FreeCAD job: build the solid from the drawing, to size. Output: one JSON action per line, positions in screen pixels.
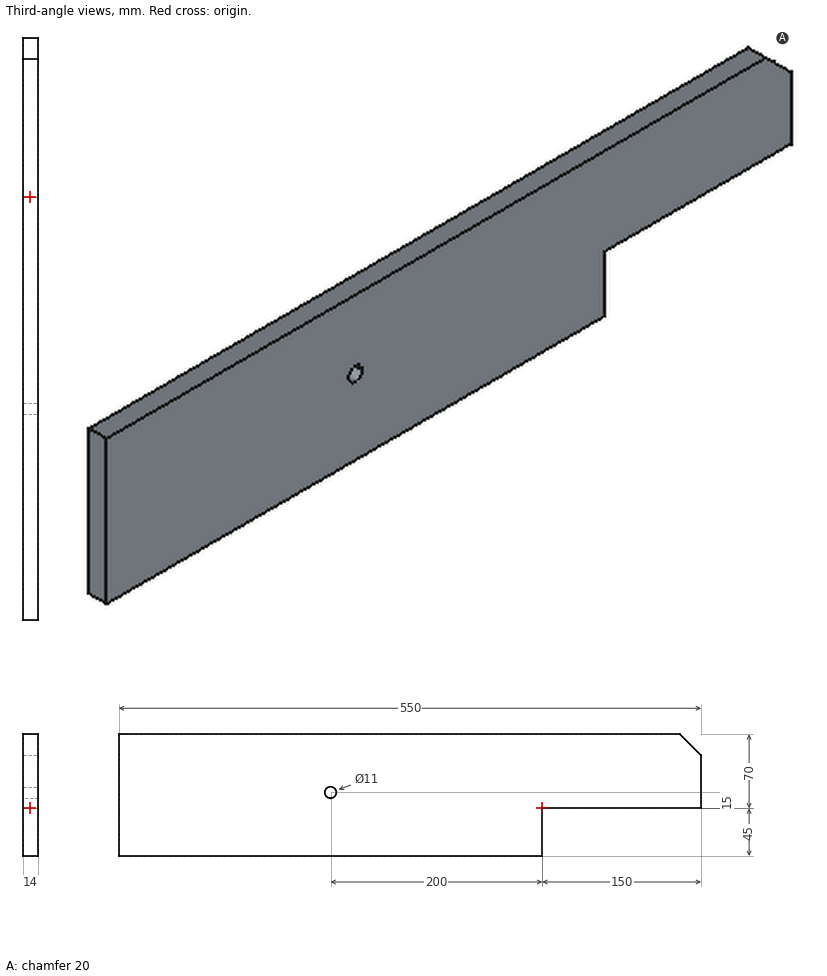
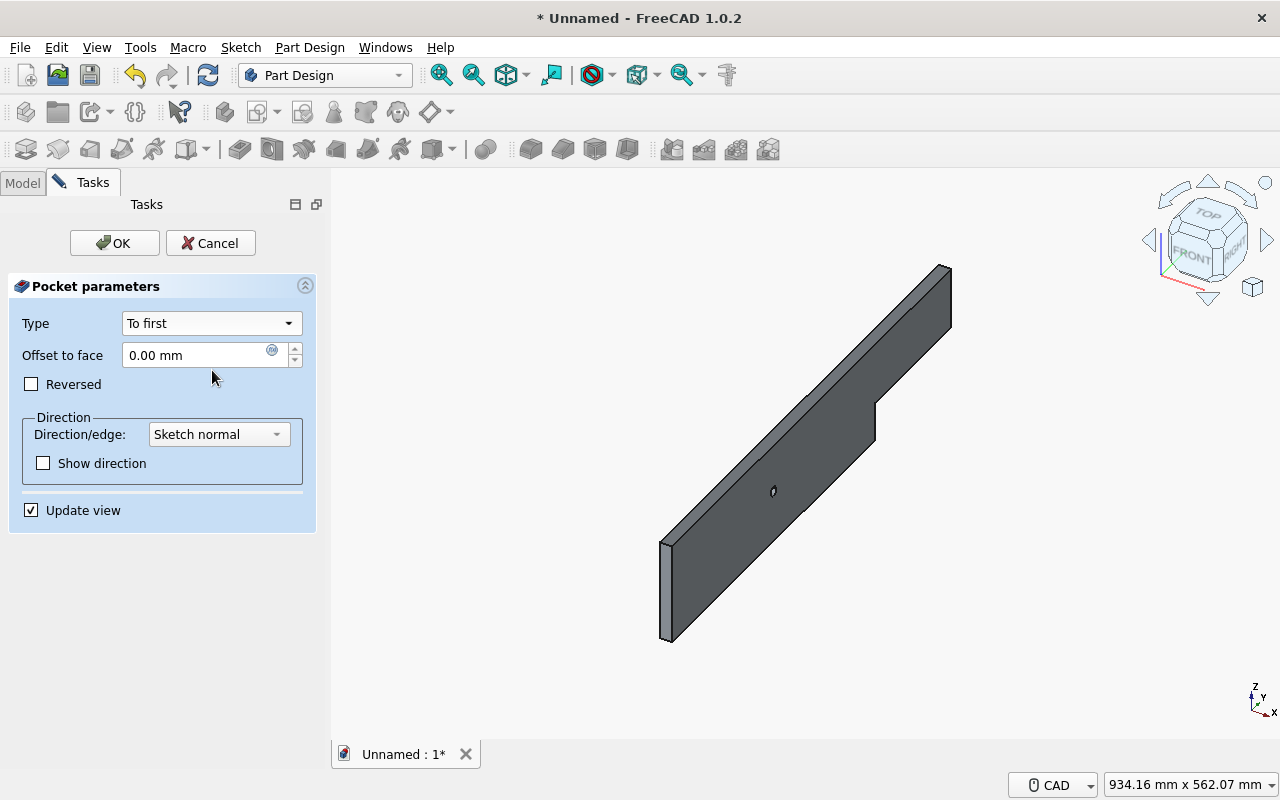
{"action": "left_click", "coordinate": [115, 243]}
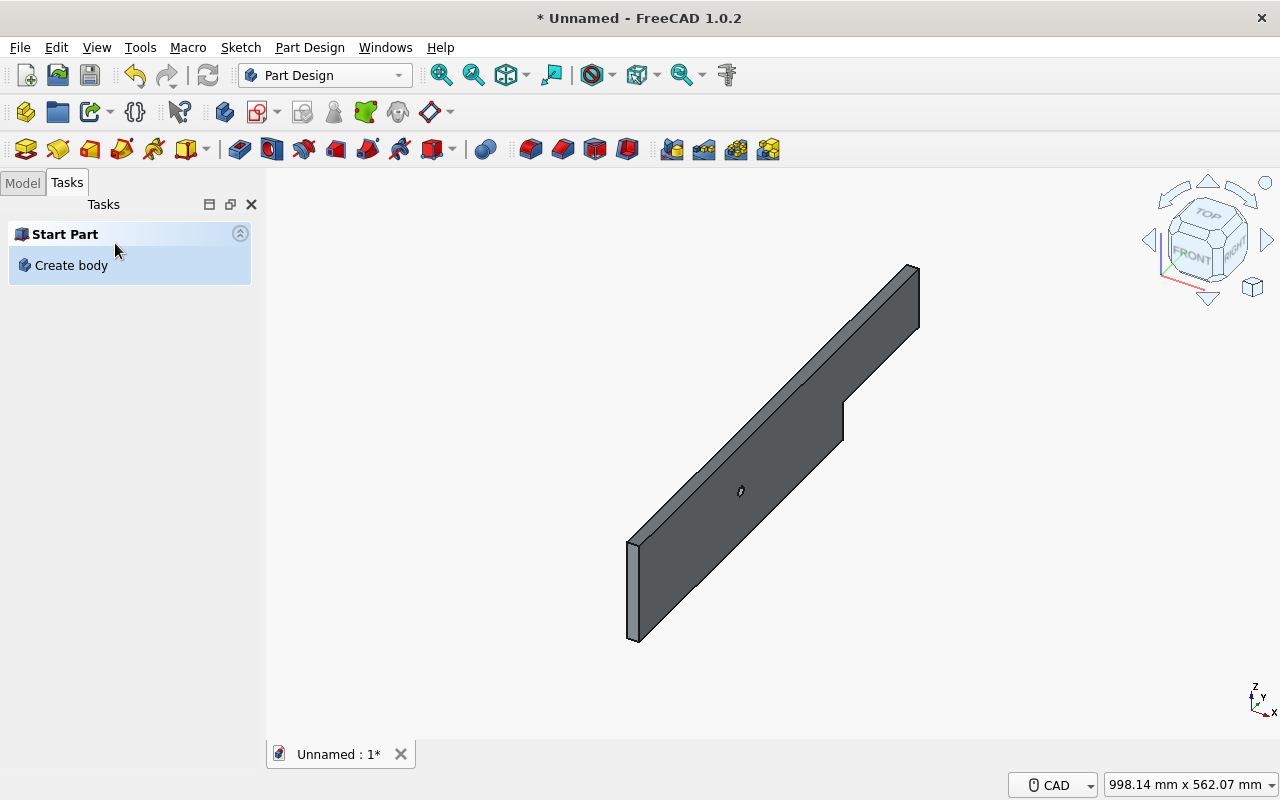
{"action": "scroll", "coordinate": [913, 266], "scroll_direction": "up", "scroll_amount": 6}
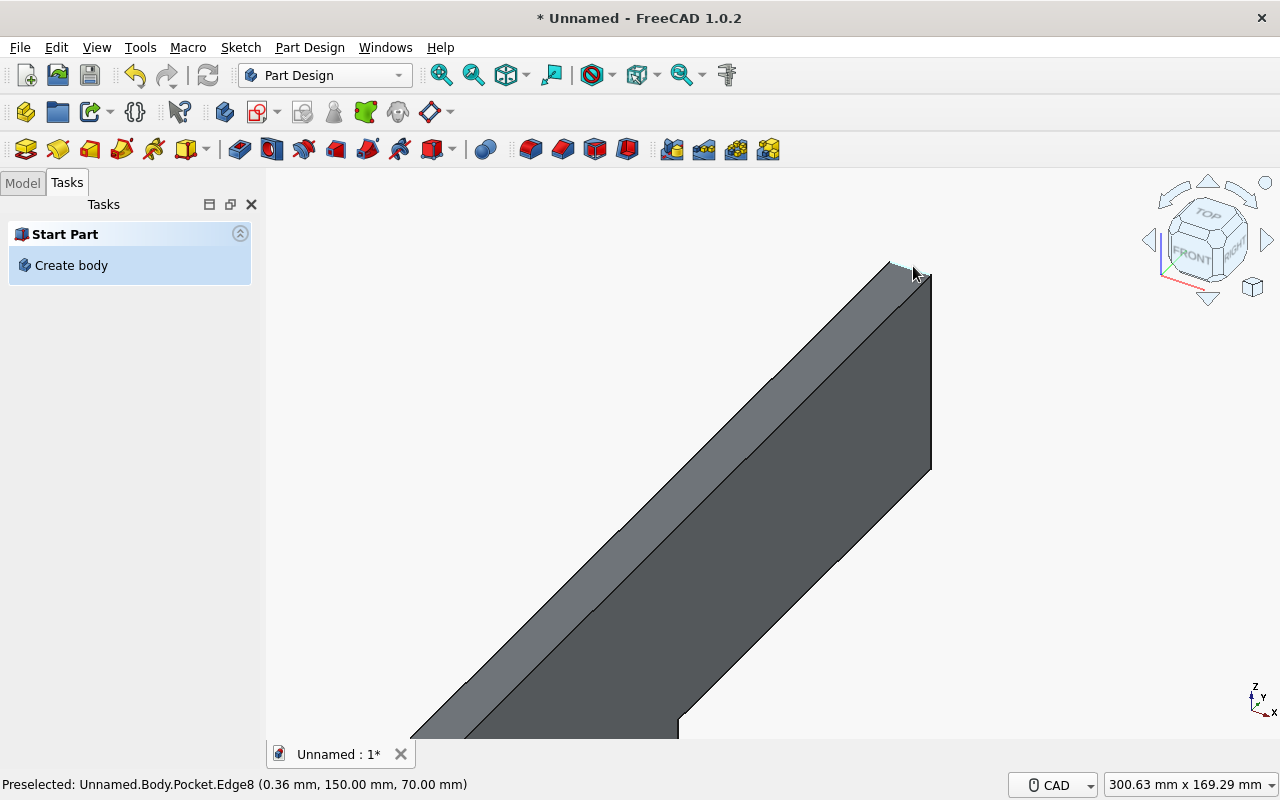
{"action": "left_click", "coordinate": [442, 76]}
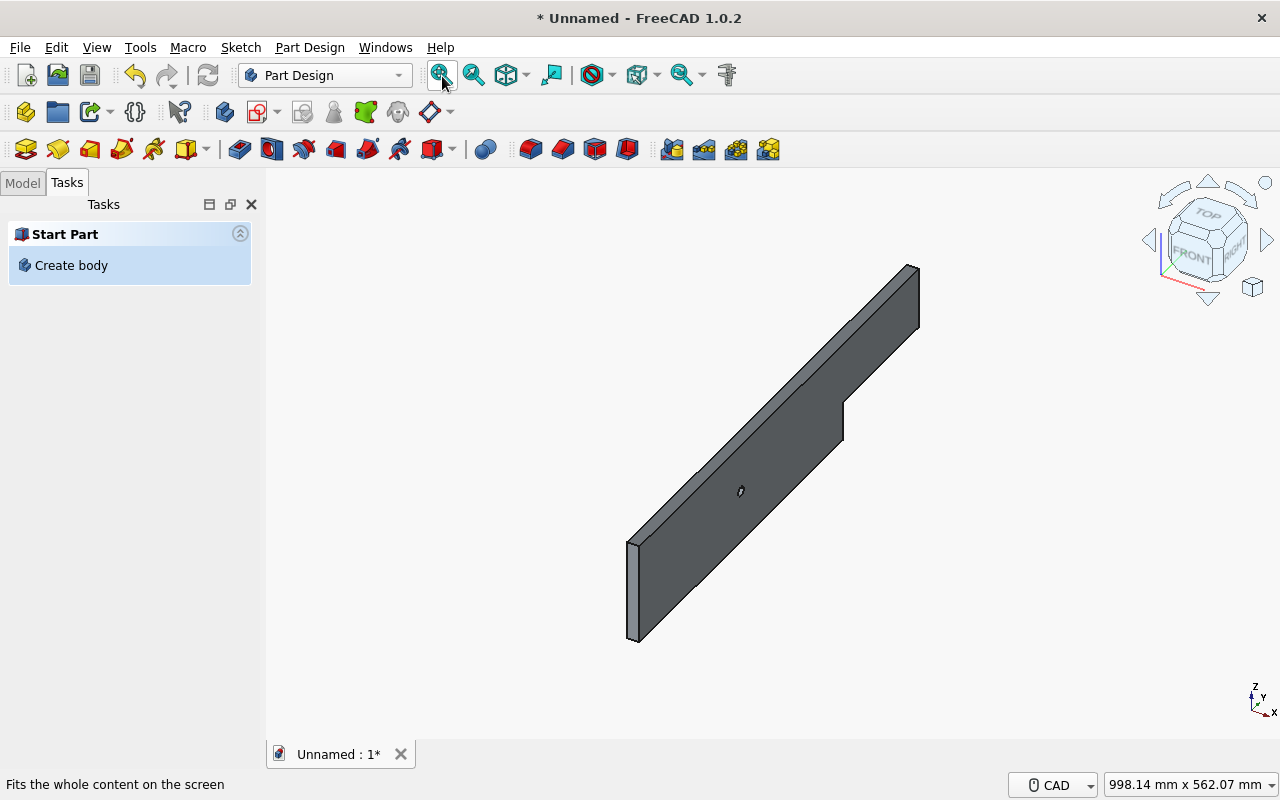
{"action": "key", "text": "0"}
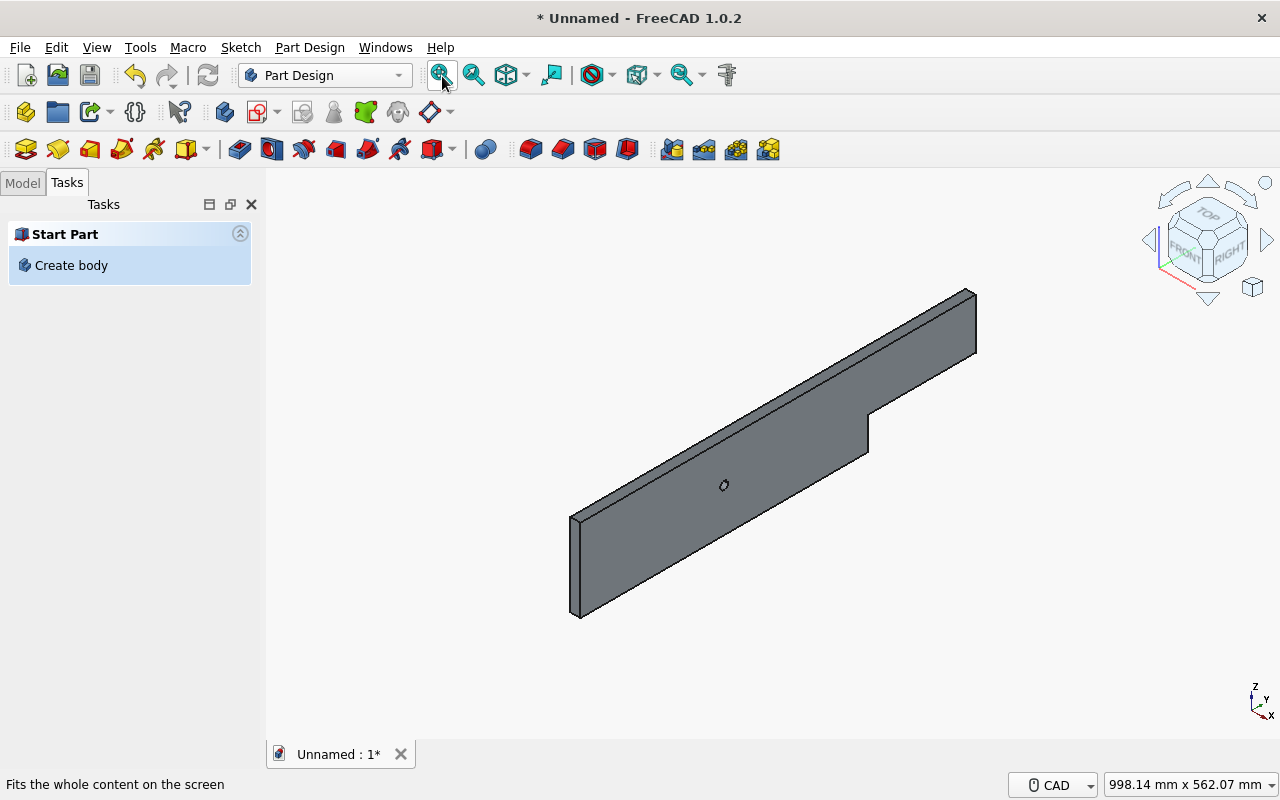
{"action": "scroll", "coordinate": [971, 291], "scroll_direction": "up", "scroll_amount": 6}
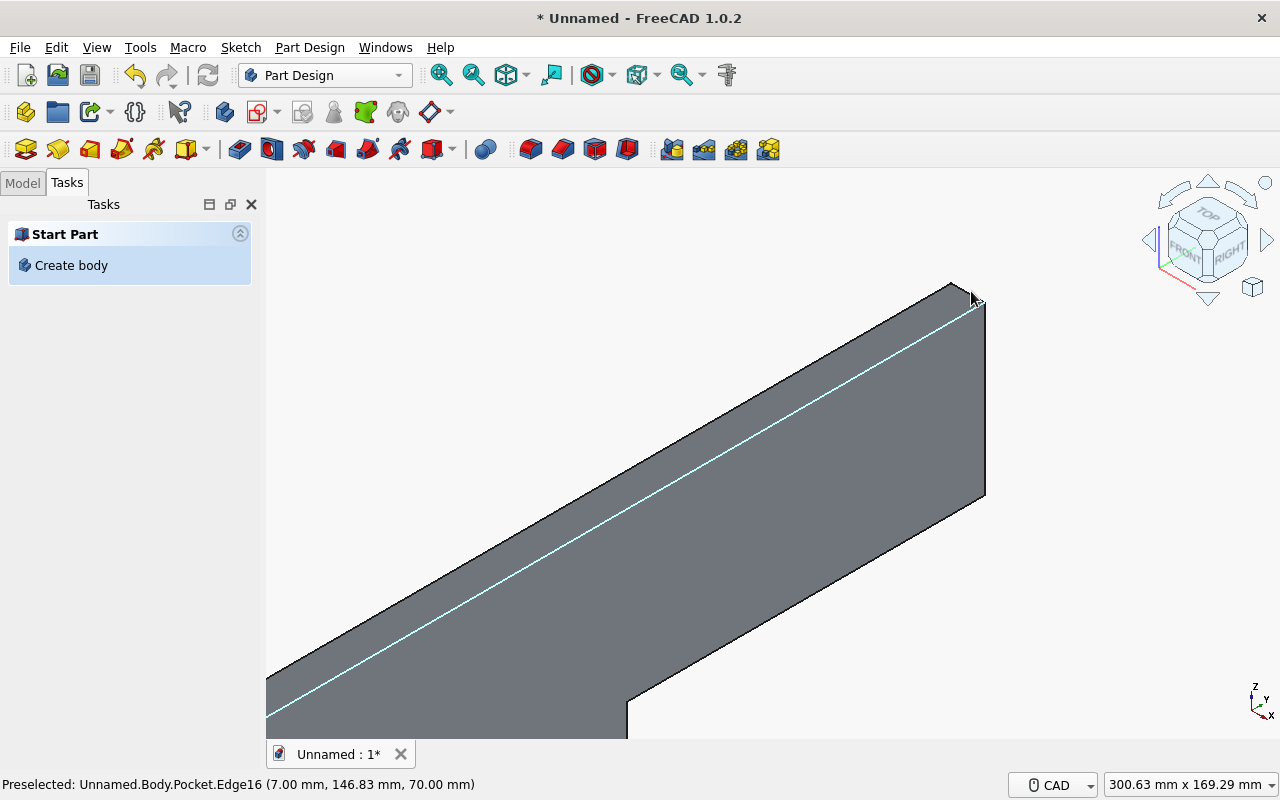
{"action": "left_click", "coordinate": [442, 76]}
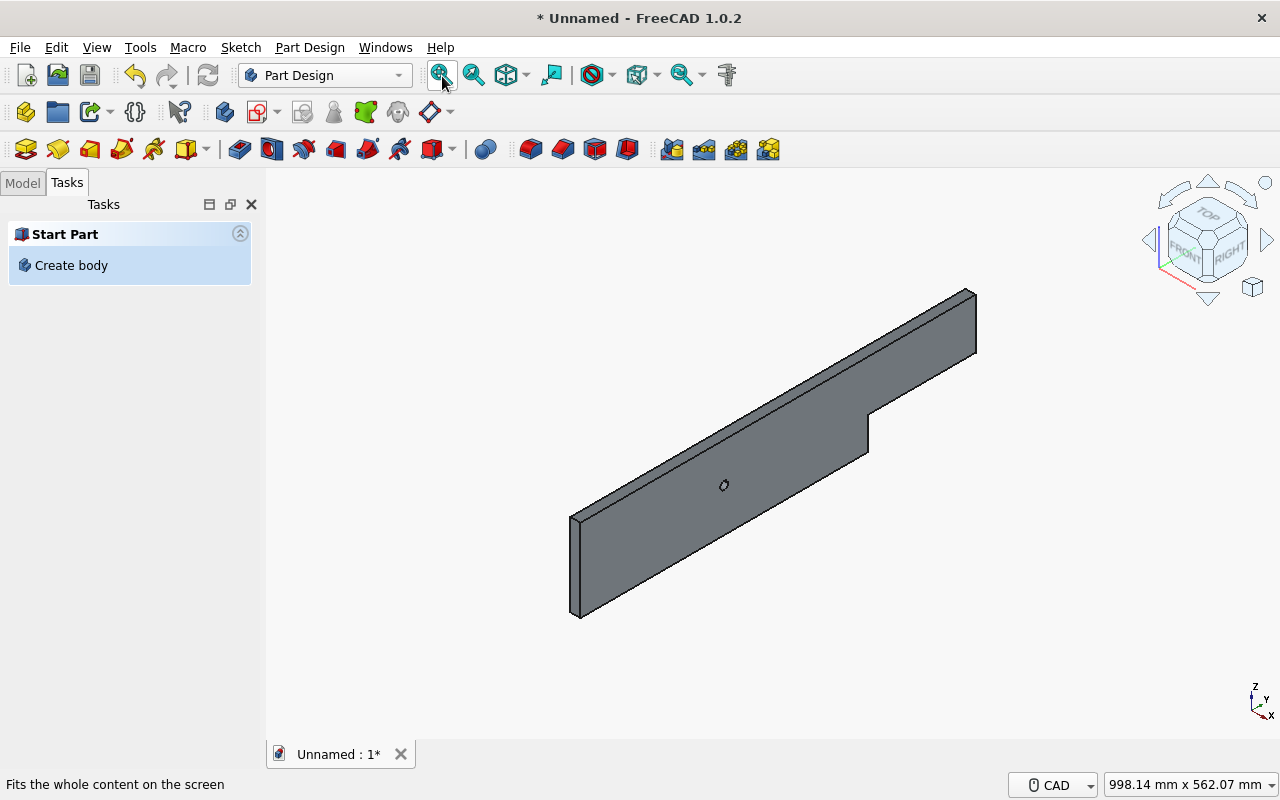
{"action": "key", "text": "2"}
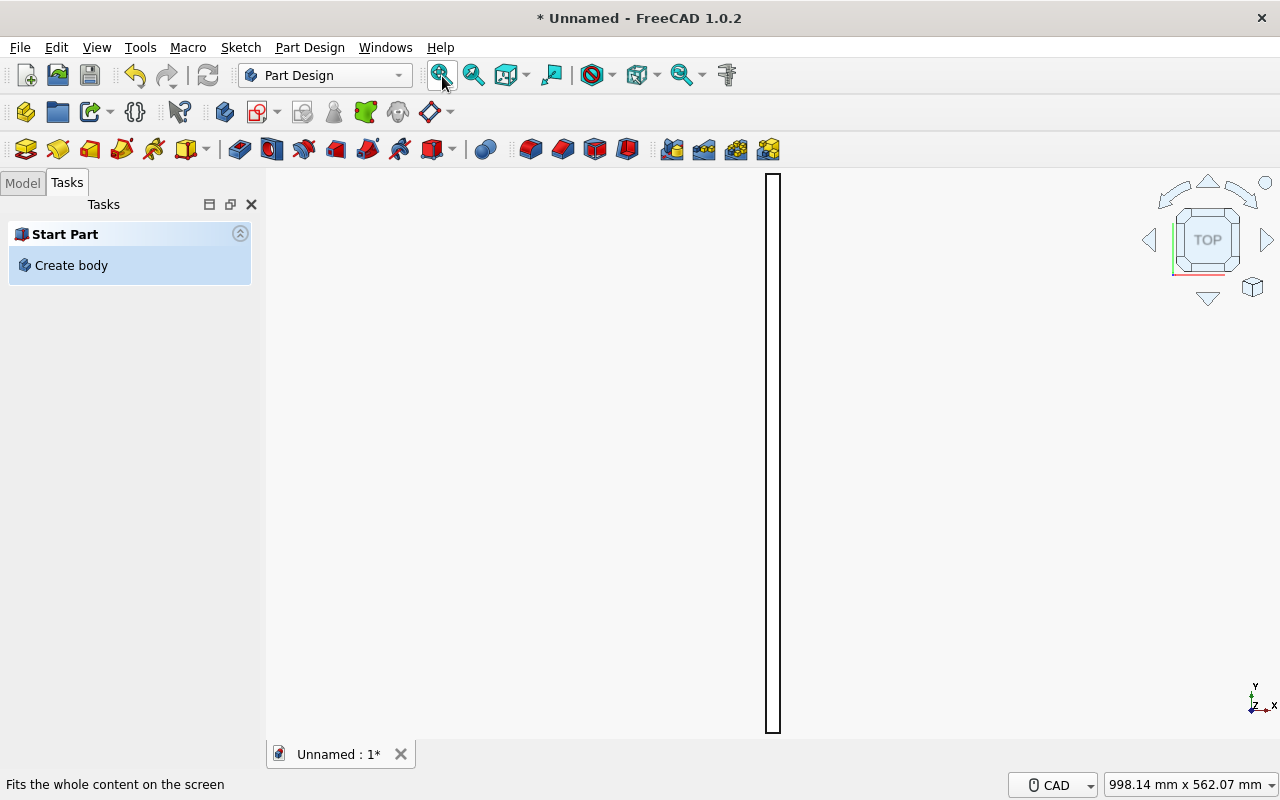
{"action": "key", "text": "1"}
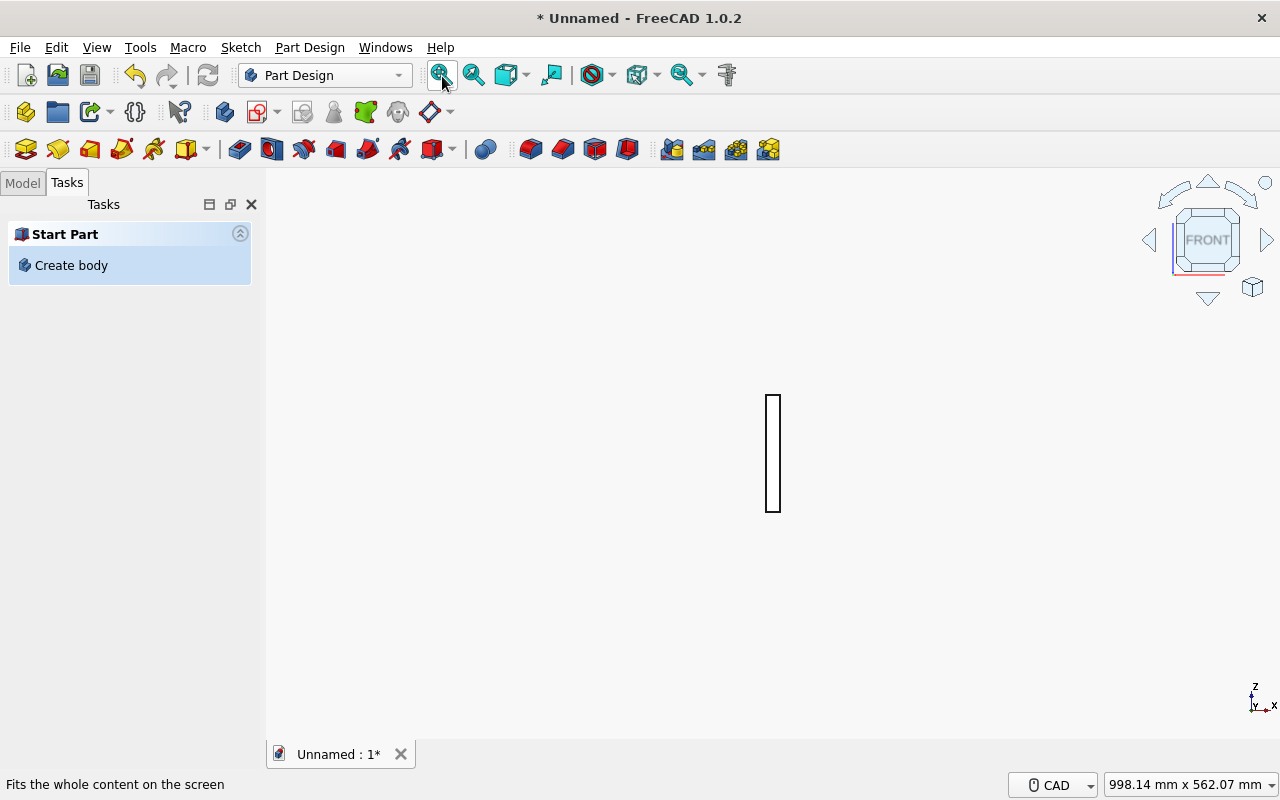
{"action": "left_click", "coordinate": [442, 76]}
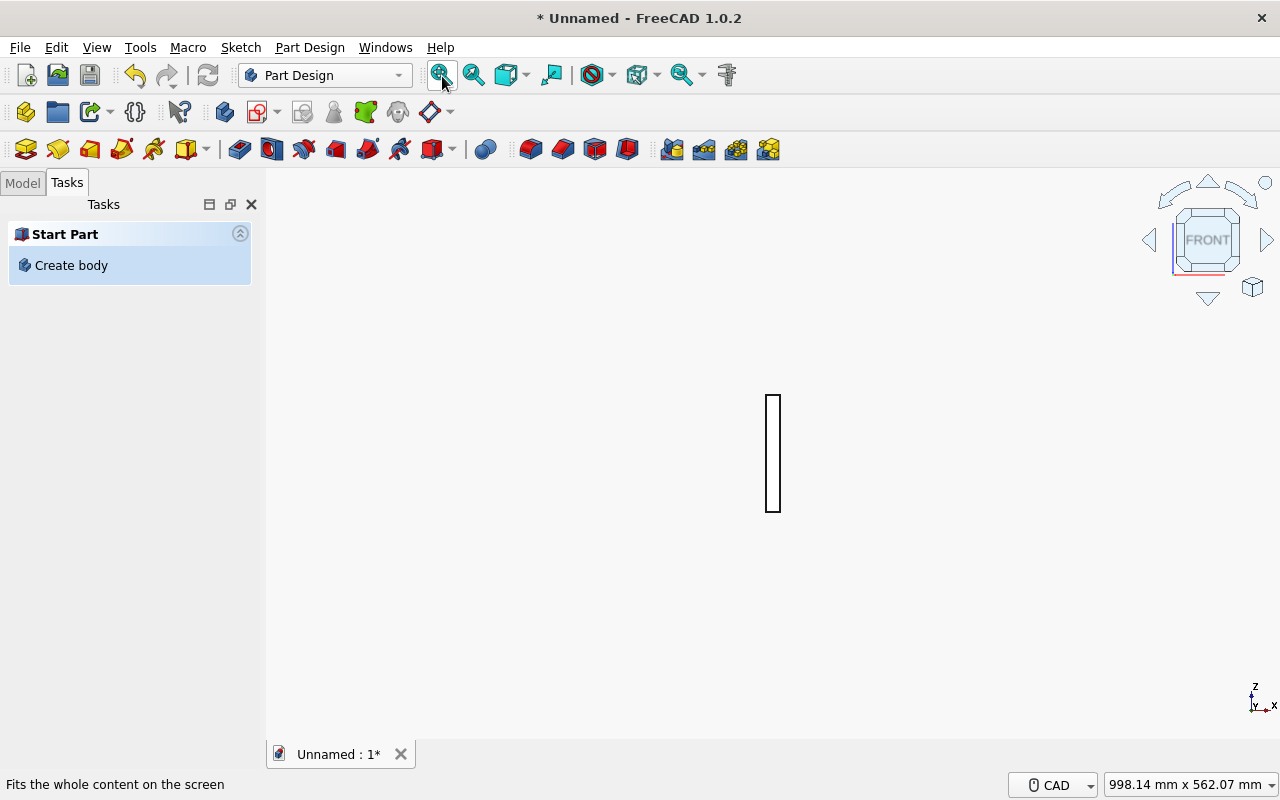
{"action": "scroll", "coordinate": [773, 394], "scroll_direction": "up", "scroll_amount": 6}